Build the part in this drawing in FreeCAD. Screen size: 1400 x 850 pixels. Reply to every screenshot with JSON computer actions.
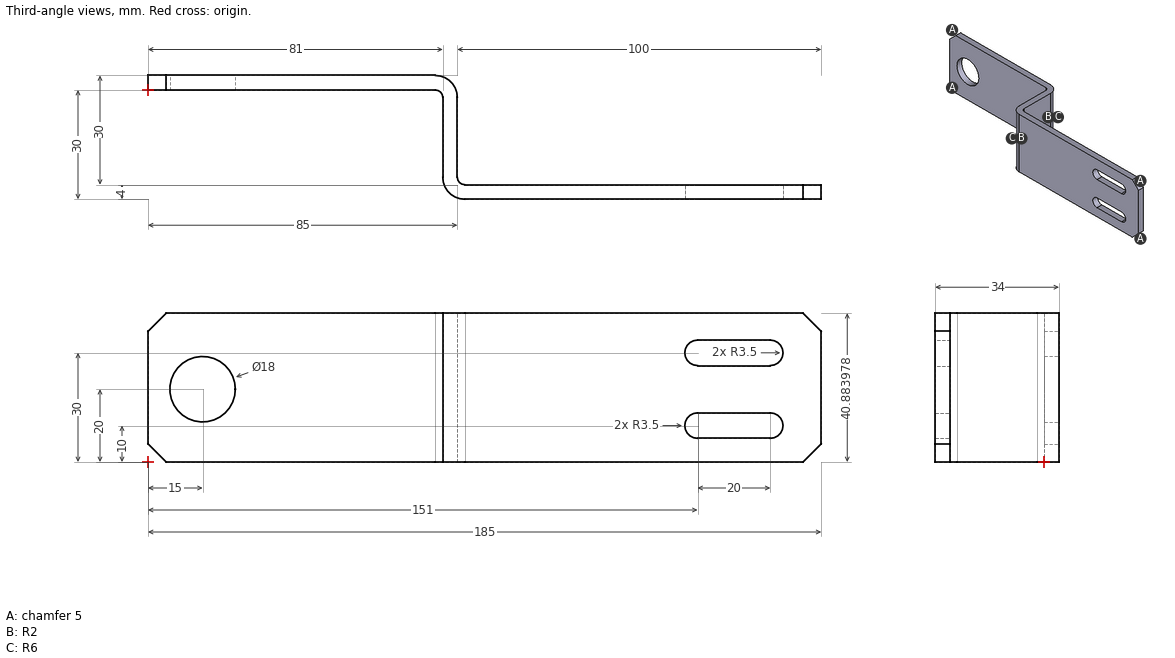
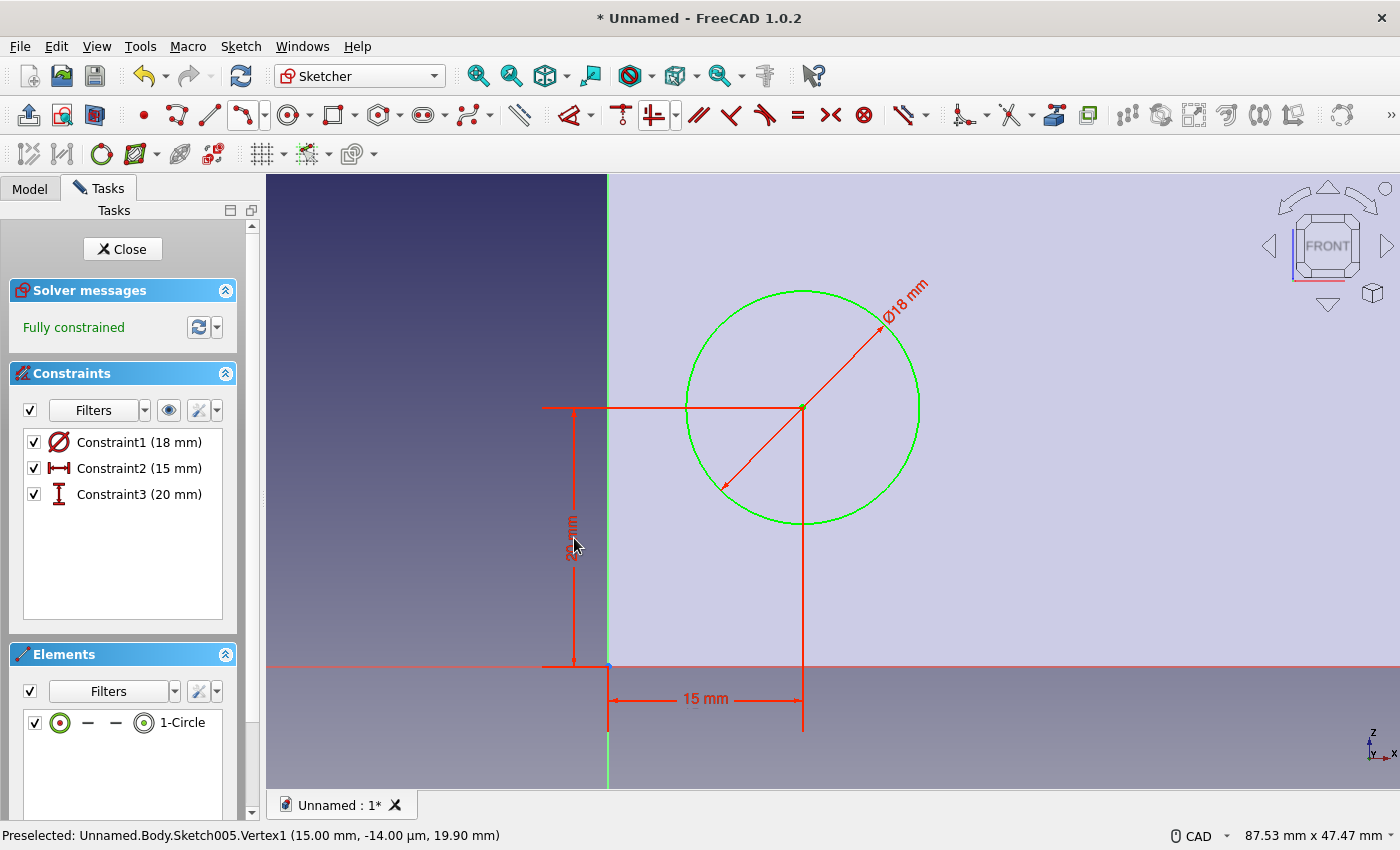
{"action": "left_click", "coordinate": [123, 249]}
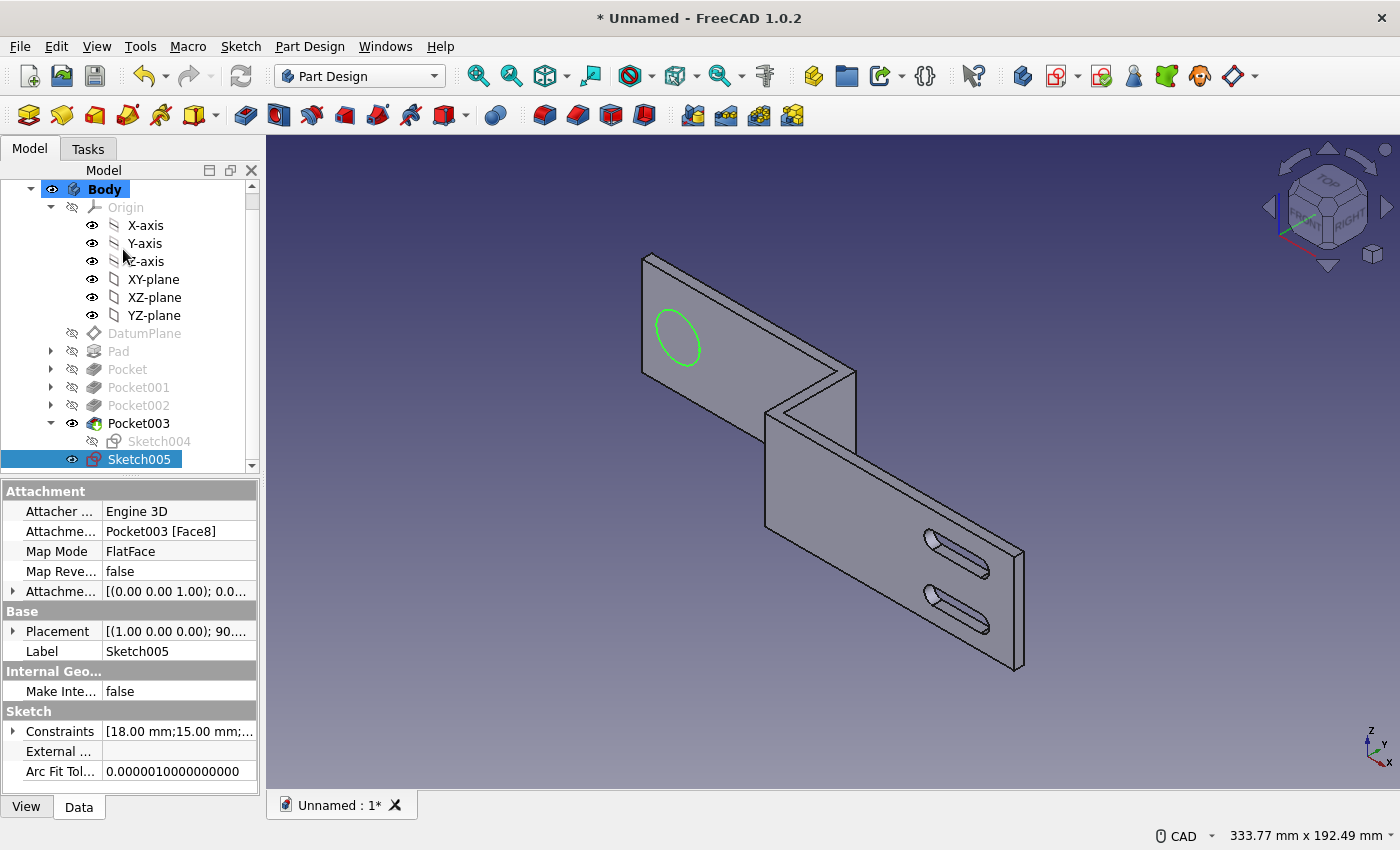
{"action": "left_click", "coordinate": [246, 116]}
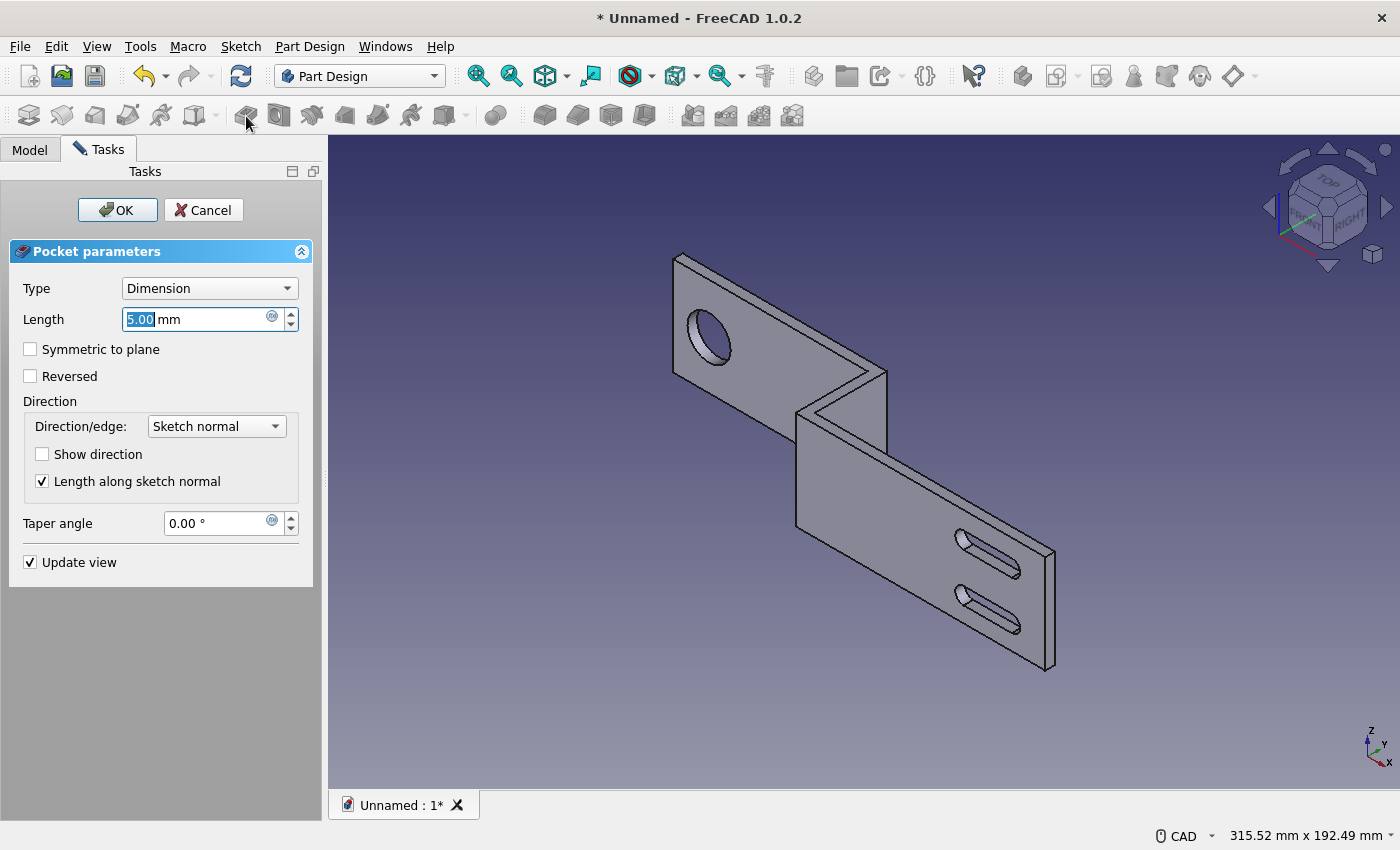
{"action": "left_click", "coordinate": [210, 288]}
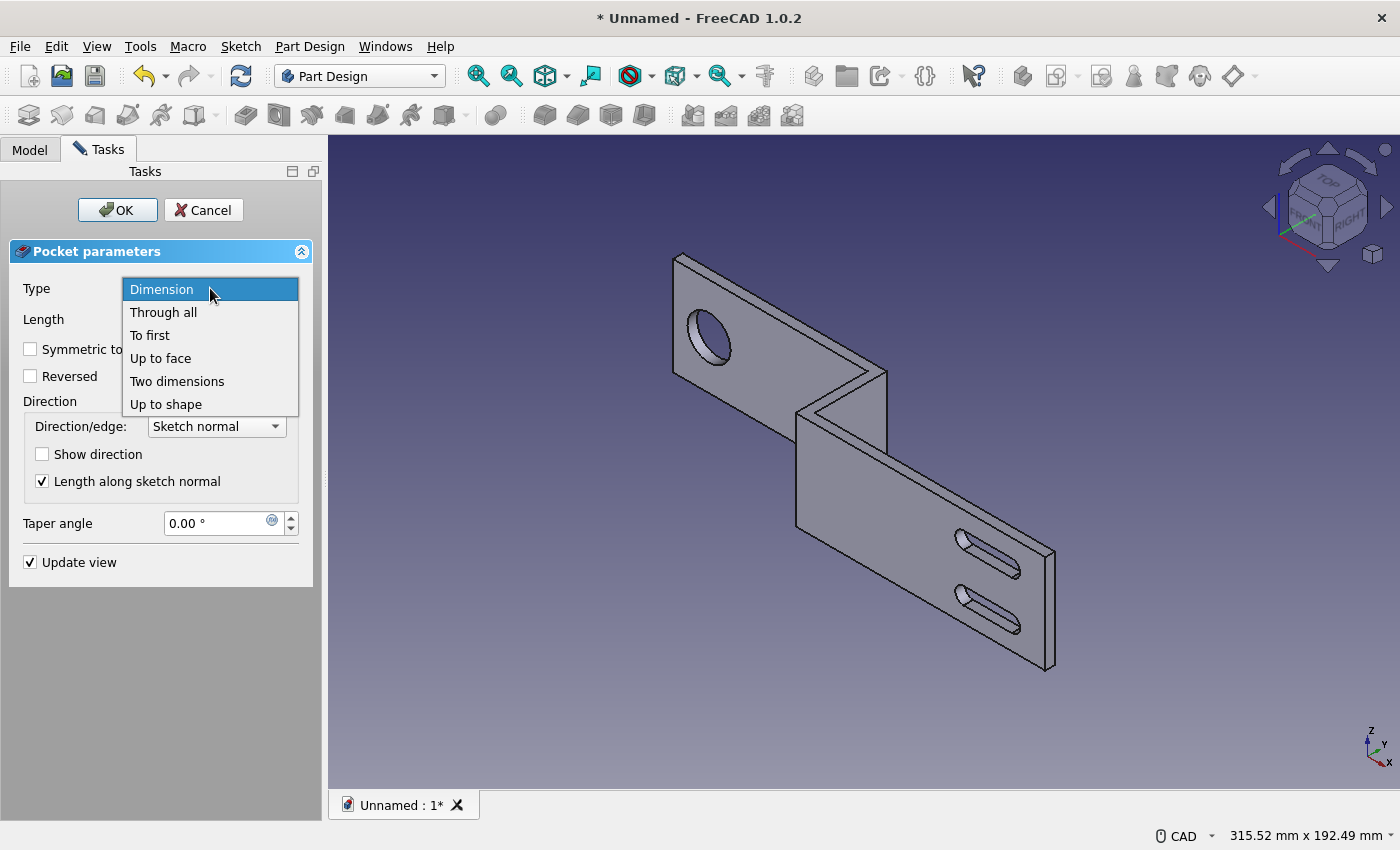
{"action": "left_click", "coordinate": [208, 312]}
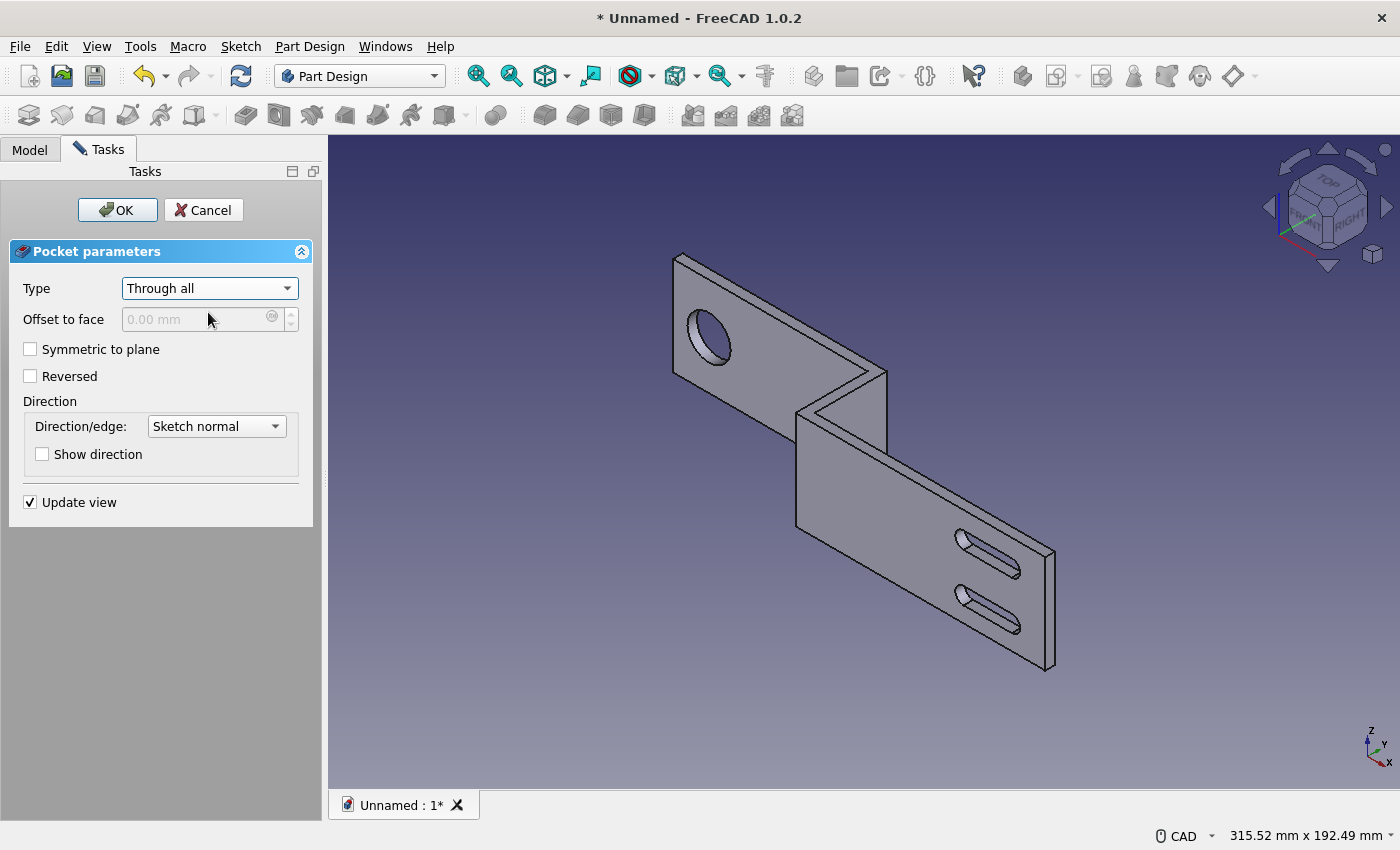
{"action": "left_click", "coordinate": [118, 210]}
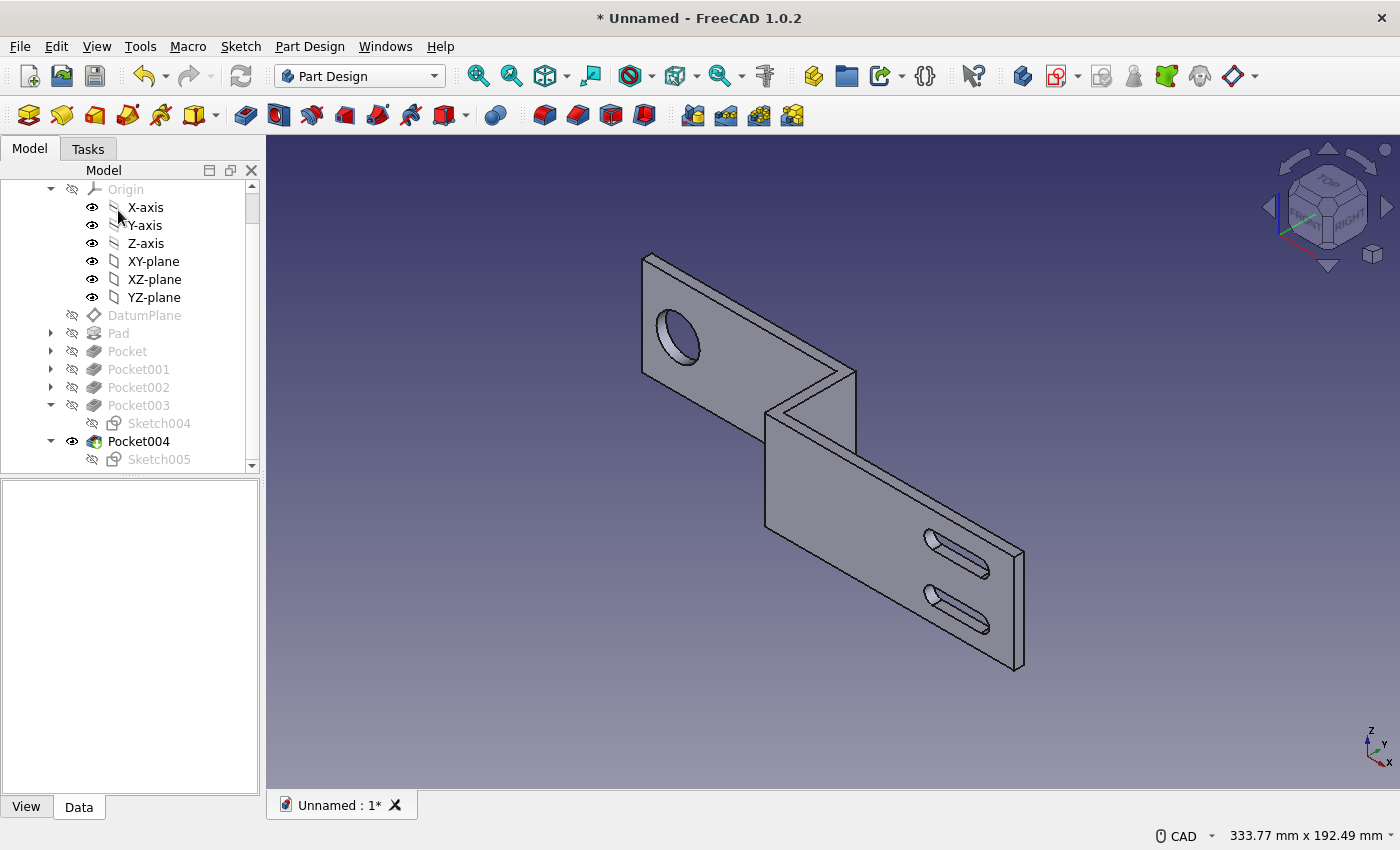
{"action": "left_click", "coordinate": [1020, 553]}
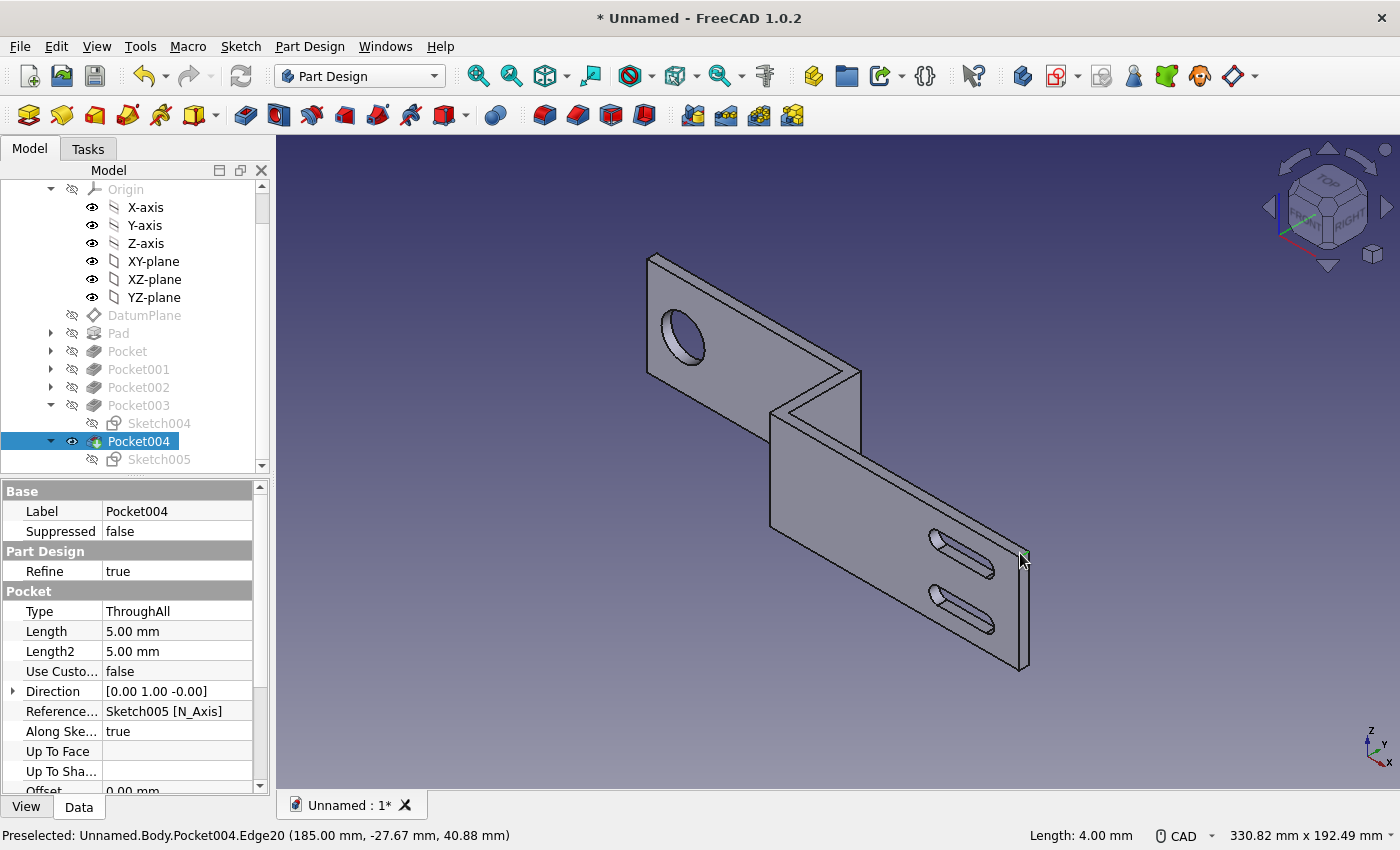
{"action": "scroll", "coordinate": [1024, 667], "scroll_direction": "up", "scroll_amount": 6}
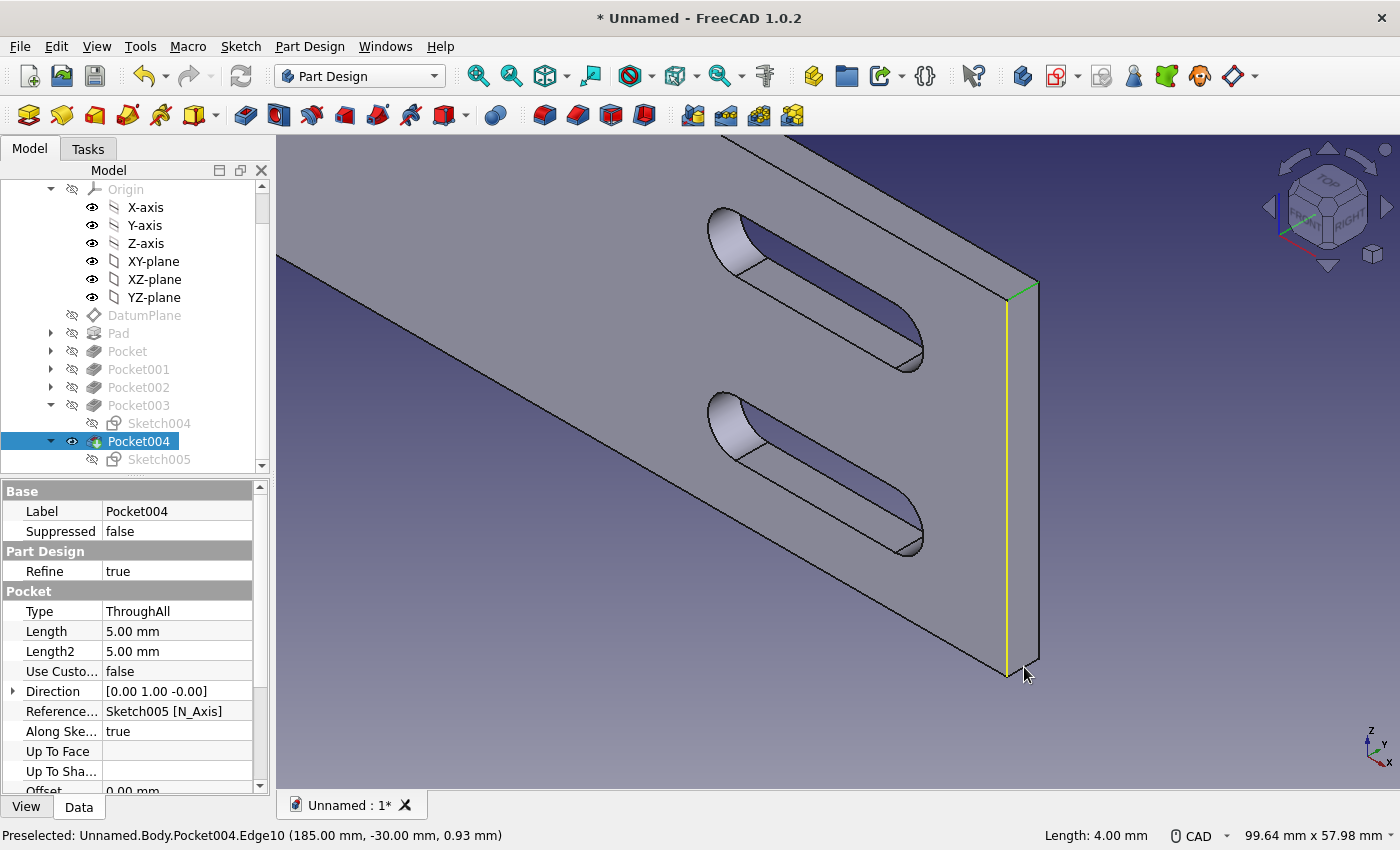
{"action": "key", "text": "v f"}